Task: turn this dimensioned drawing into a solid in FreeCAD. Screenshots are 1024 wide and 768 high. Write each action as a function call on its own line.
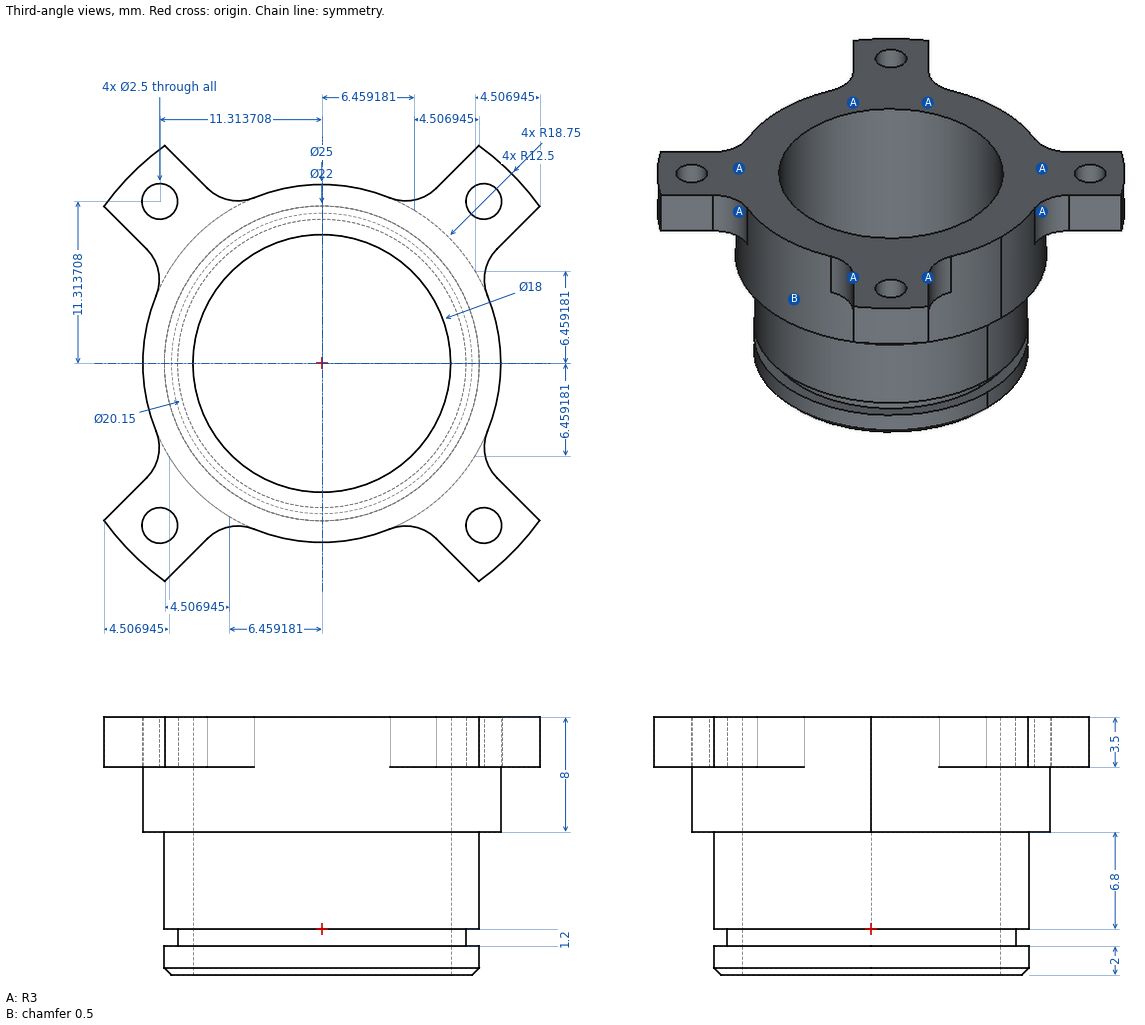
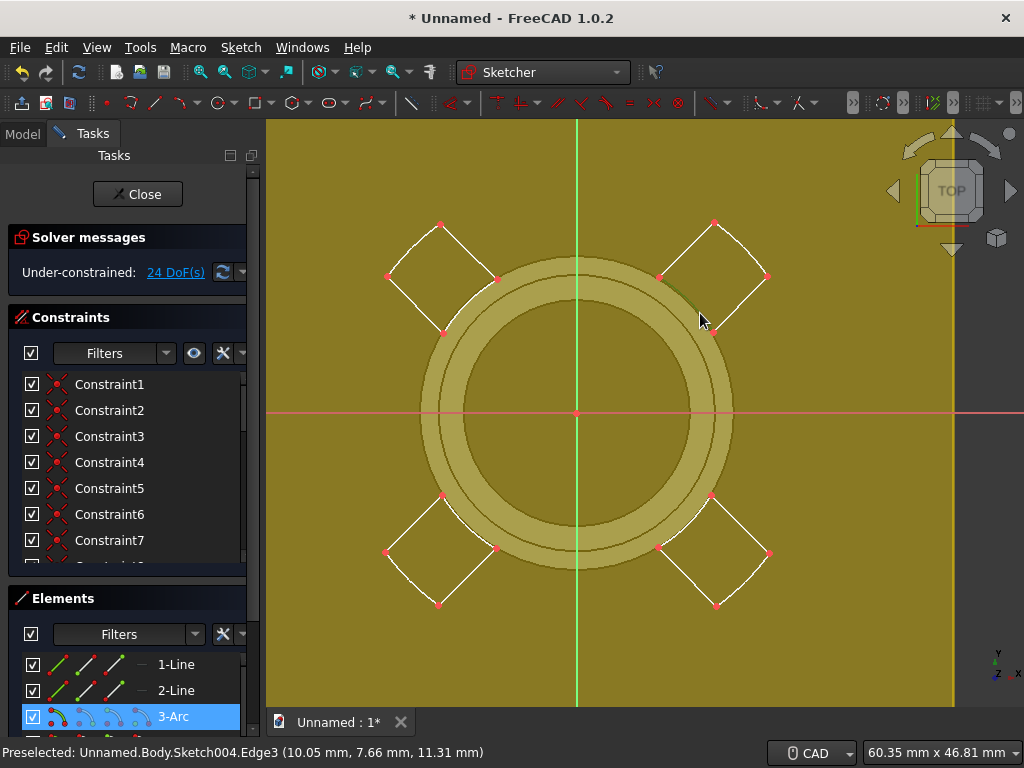
click(677, 535)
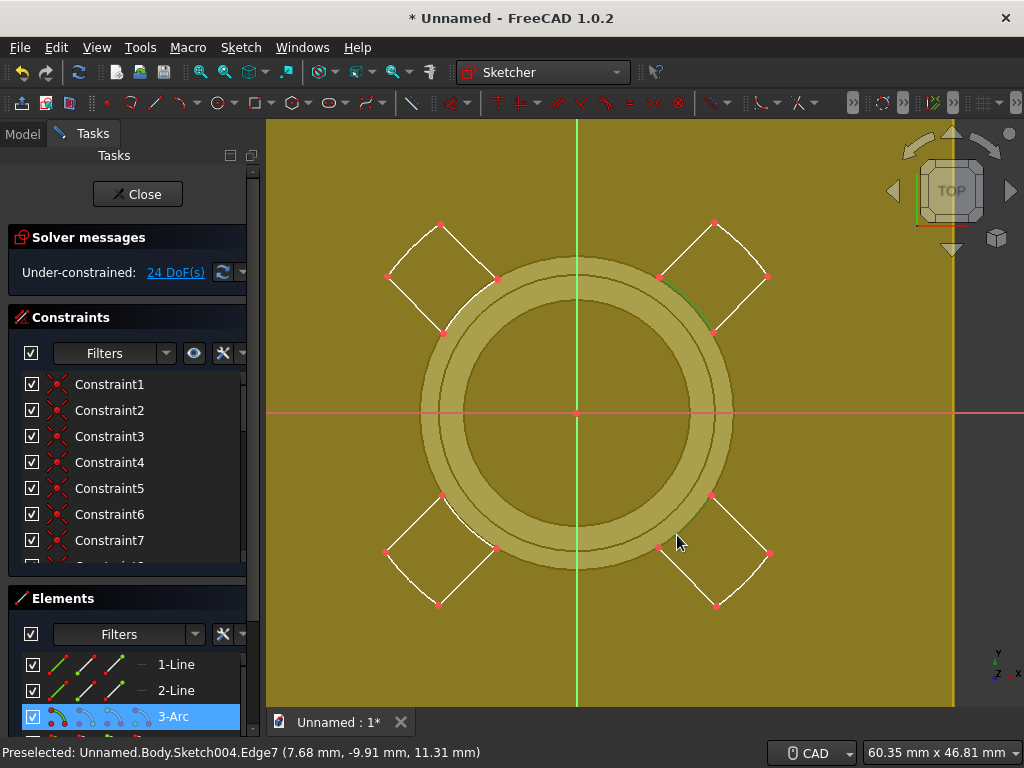
click(455, 514)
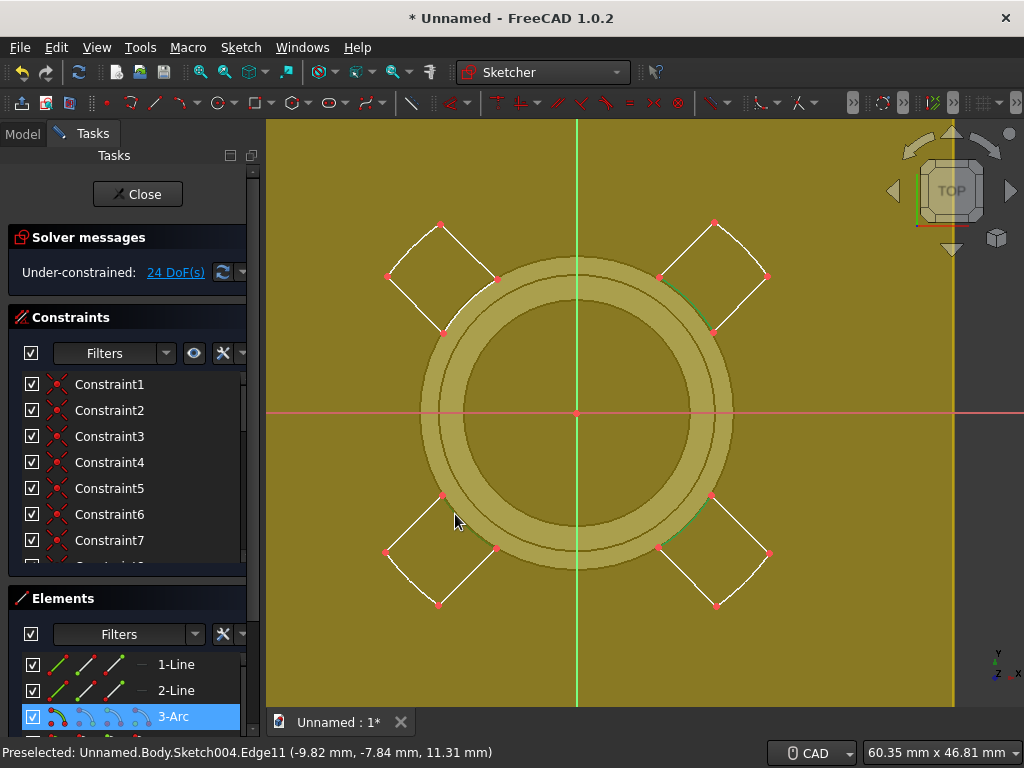
click(478, 293)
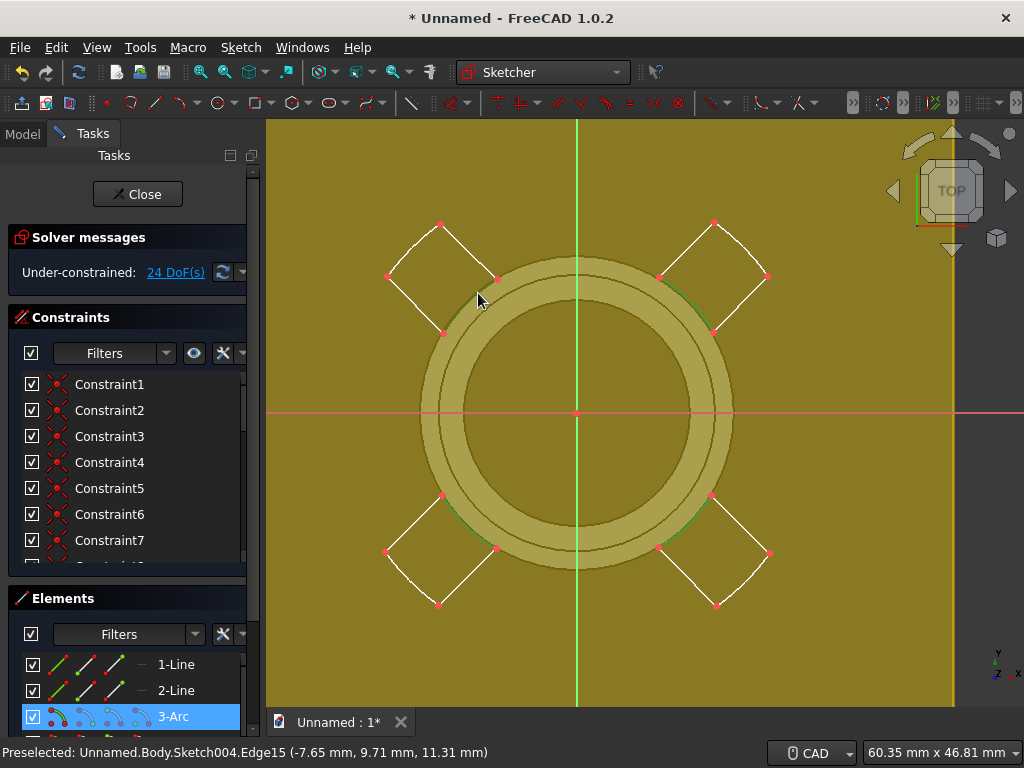
click(630, 104)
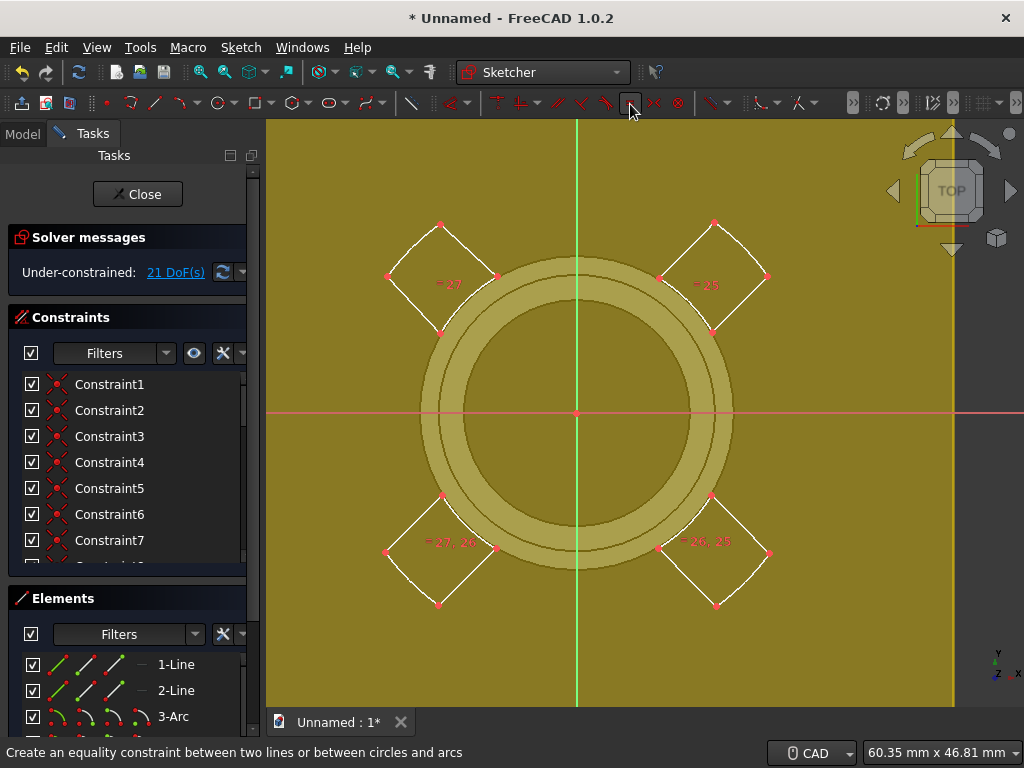
click(754, 258)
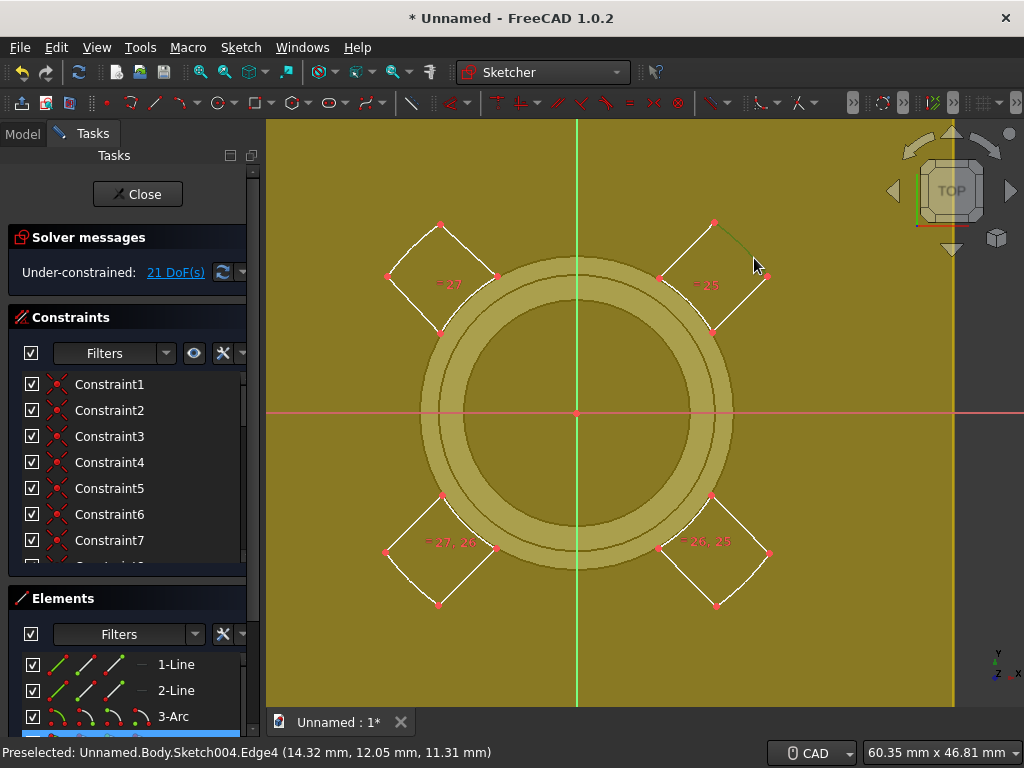
click(734, 593)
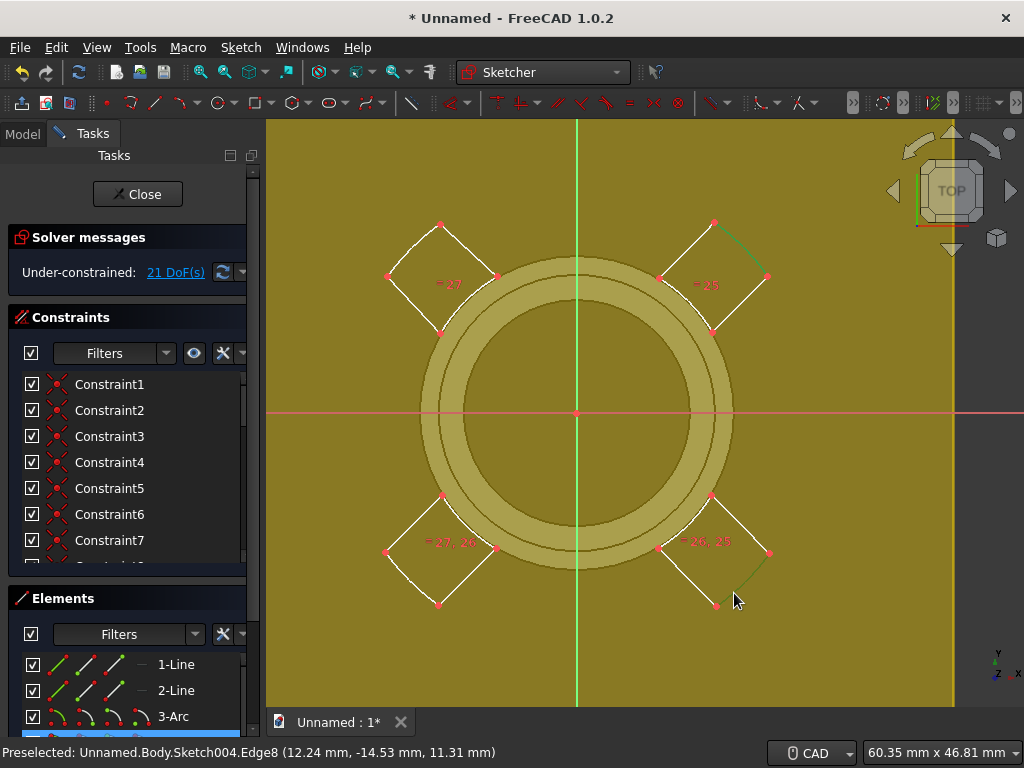
click(400, 570)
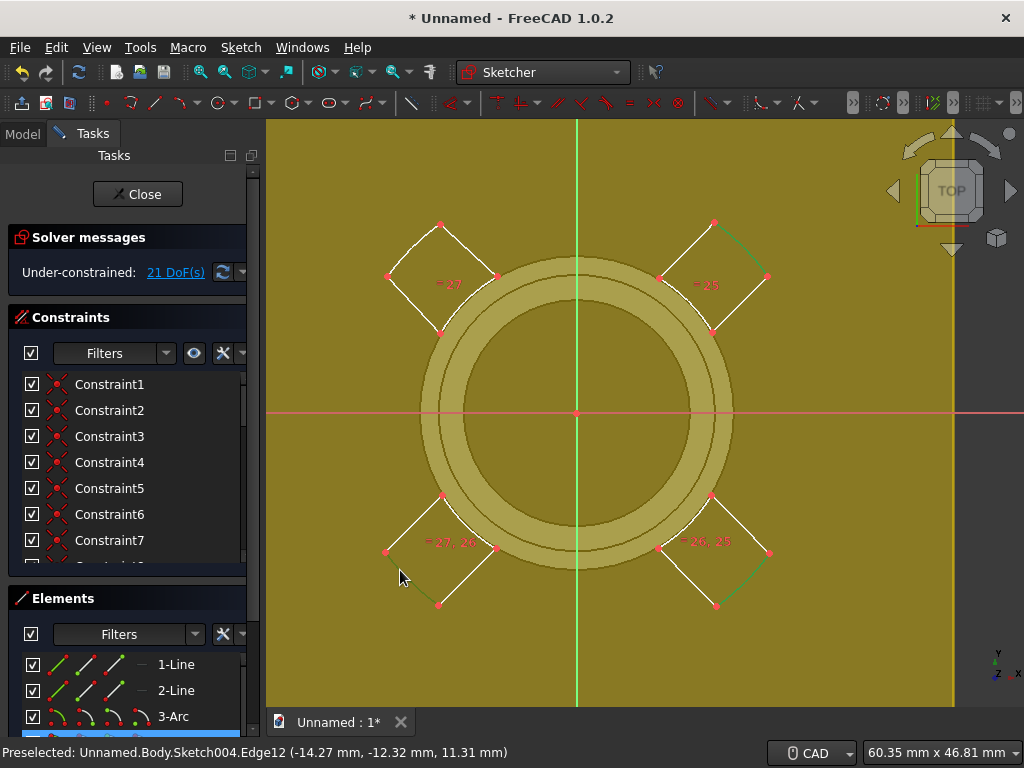
click(423, 238)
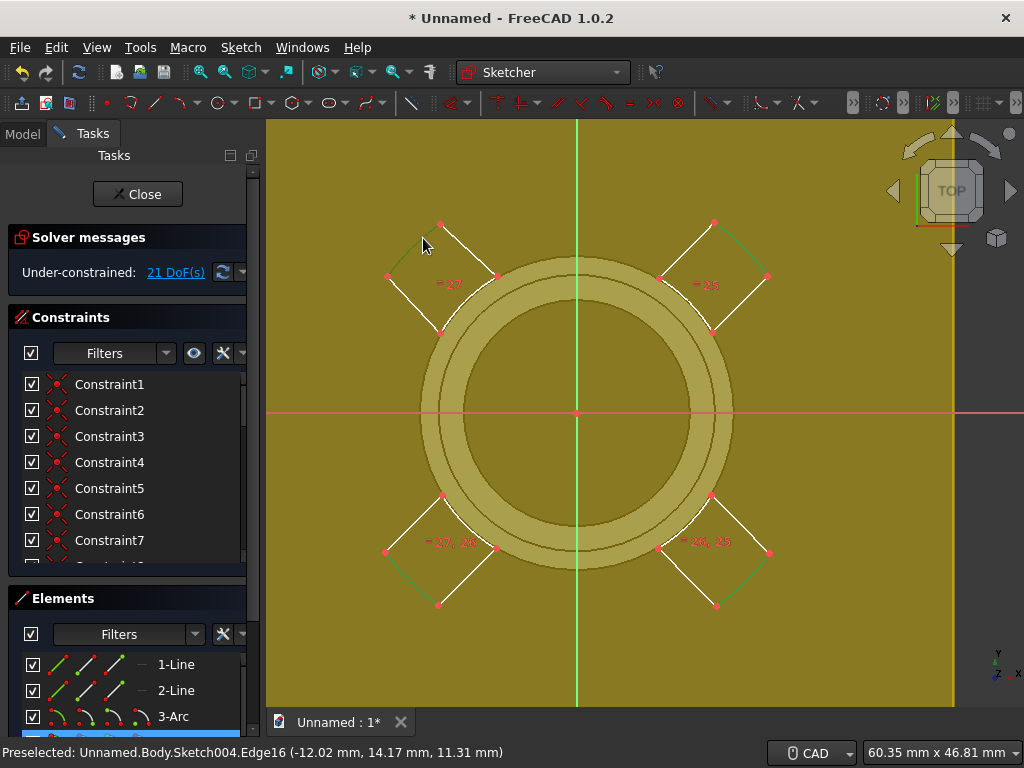
click(630, 104)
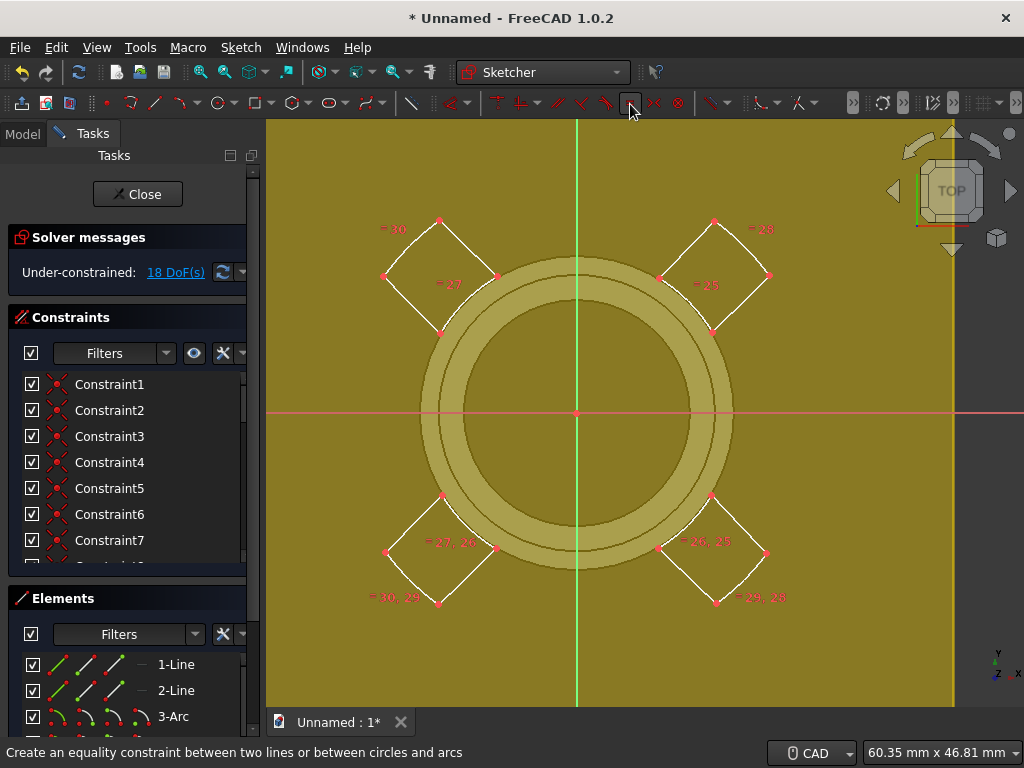
click(450, 104)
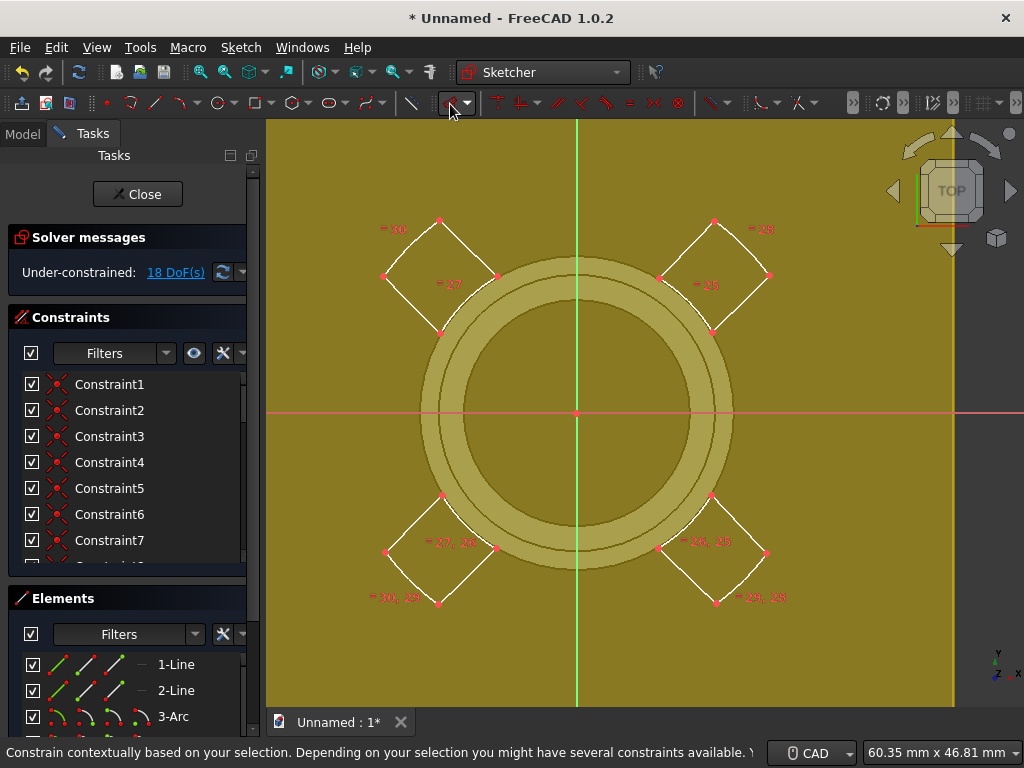
click(699, 314)
click(724, 294)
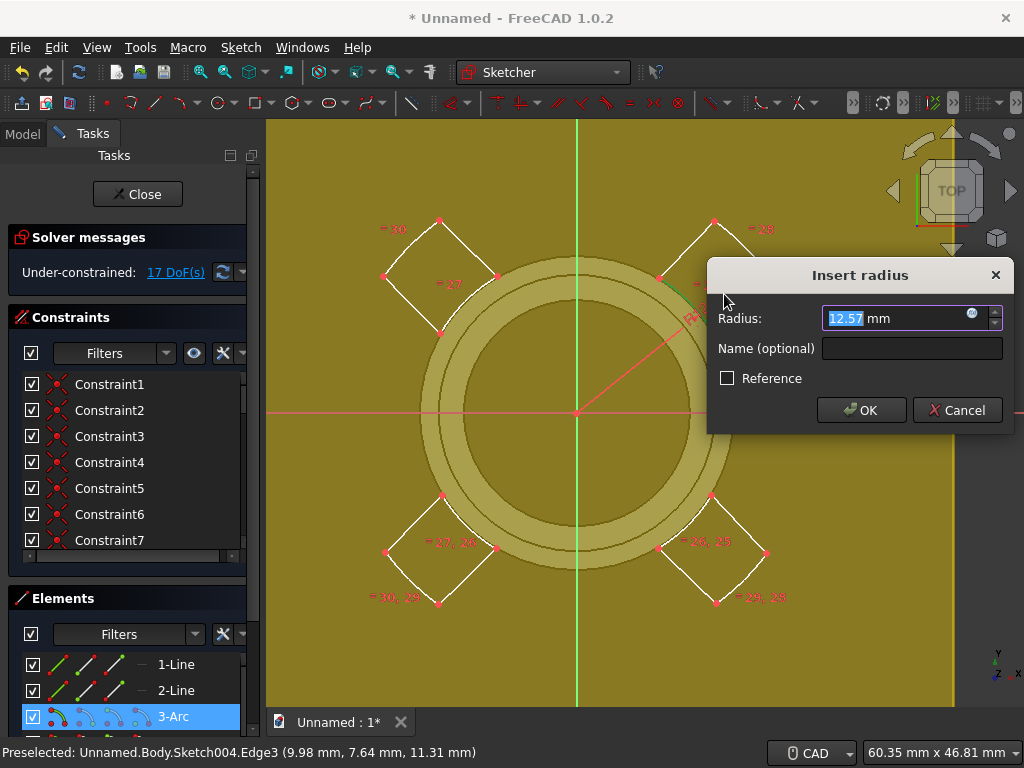
text(12.5)
key(Return)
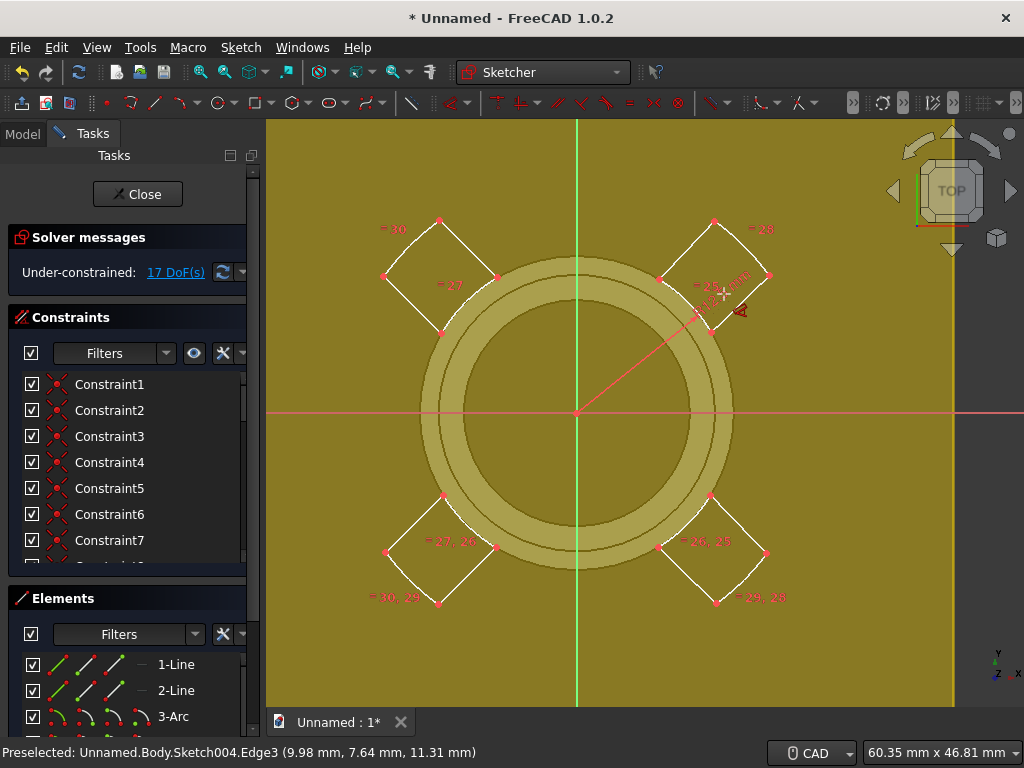
click(755, 258)
click(779, 237)